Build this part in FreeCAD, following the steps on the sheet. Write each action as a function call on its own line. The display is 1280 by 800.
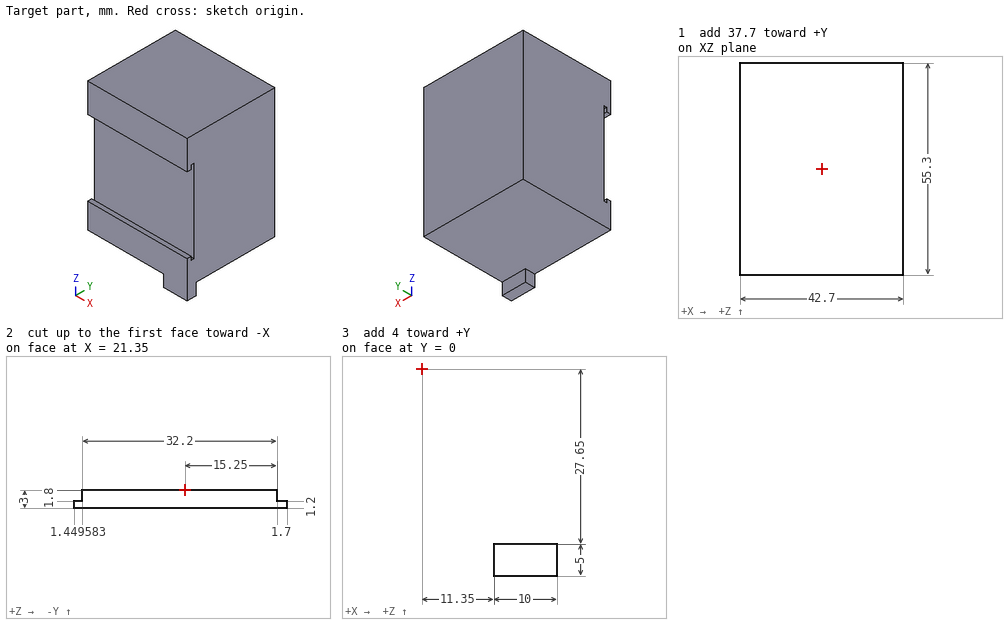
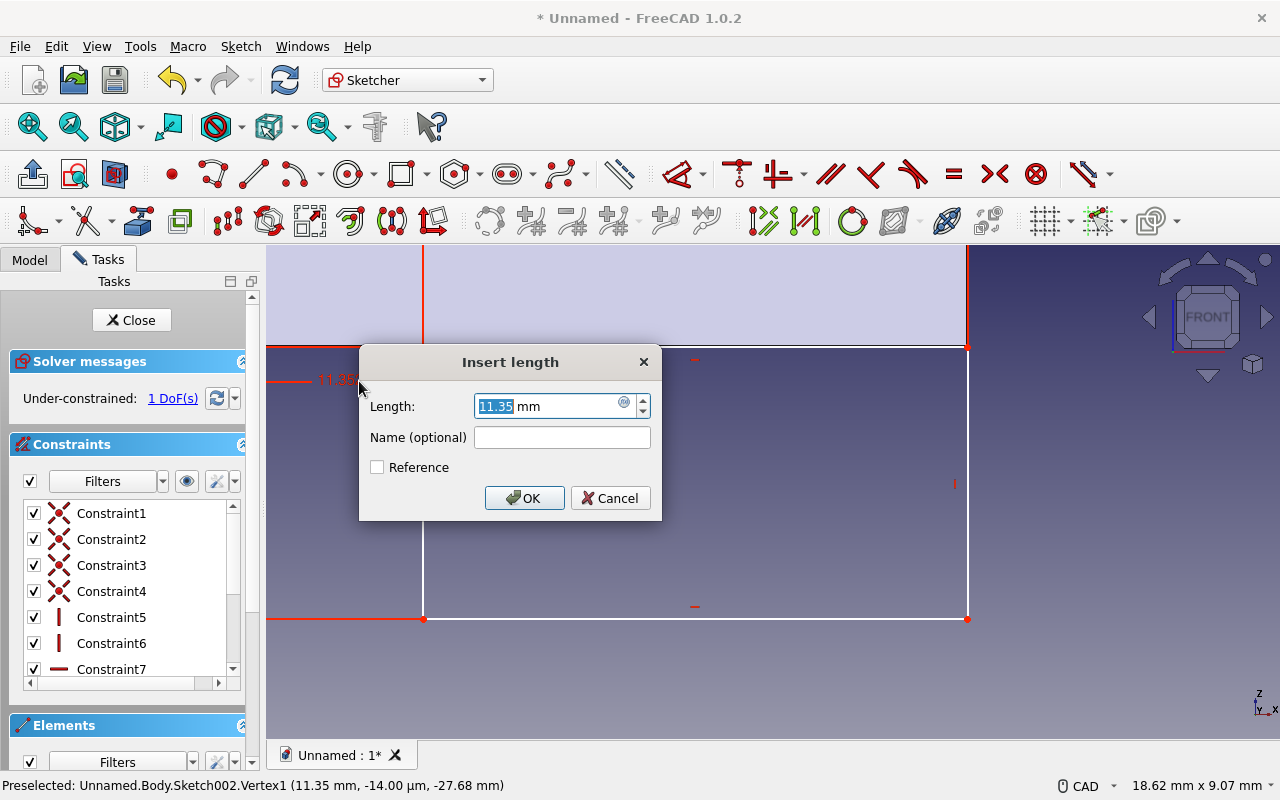
text(11.35)
key(Return)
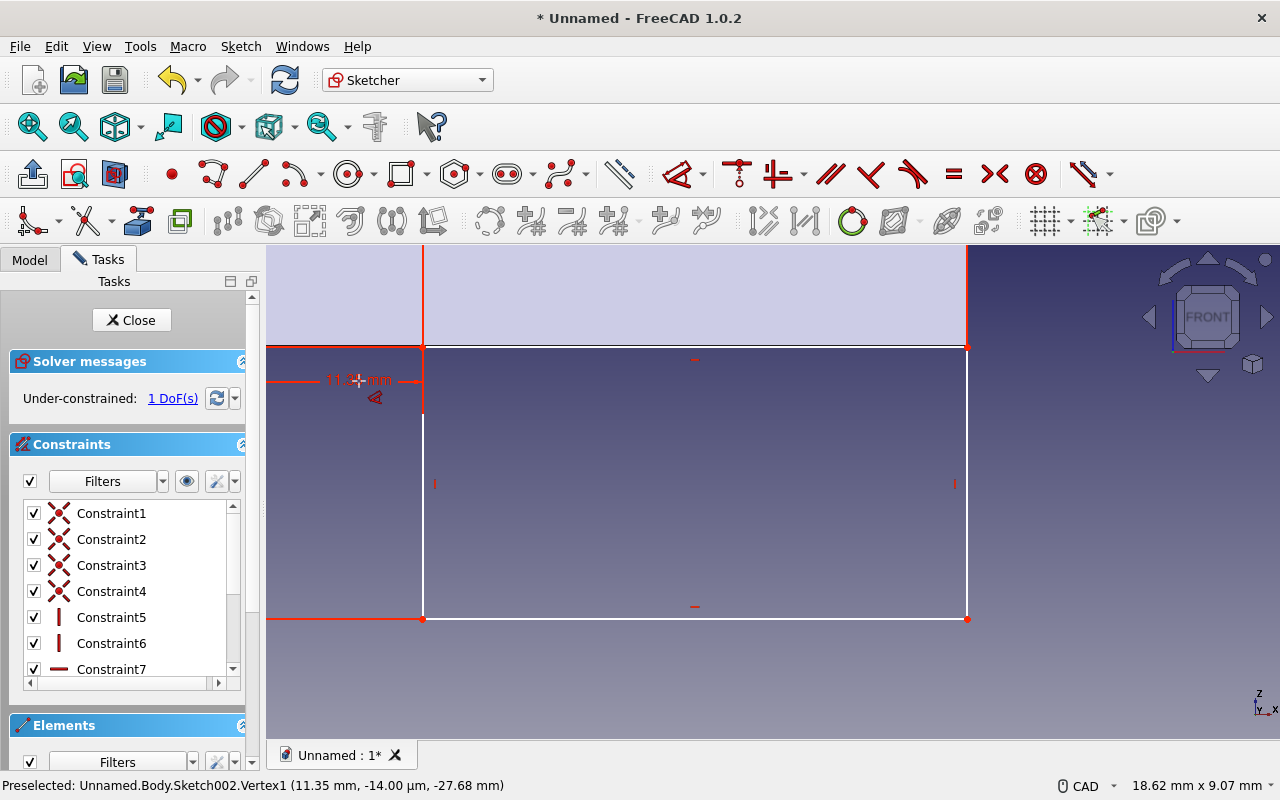
click(423, 347)
click(457, 310)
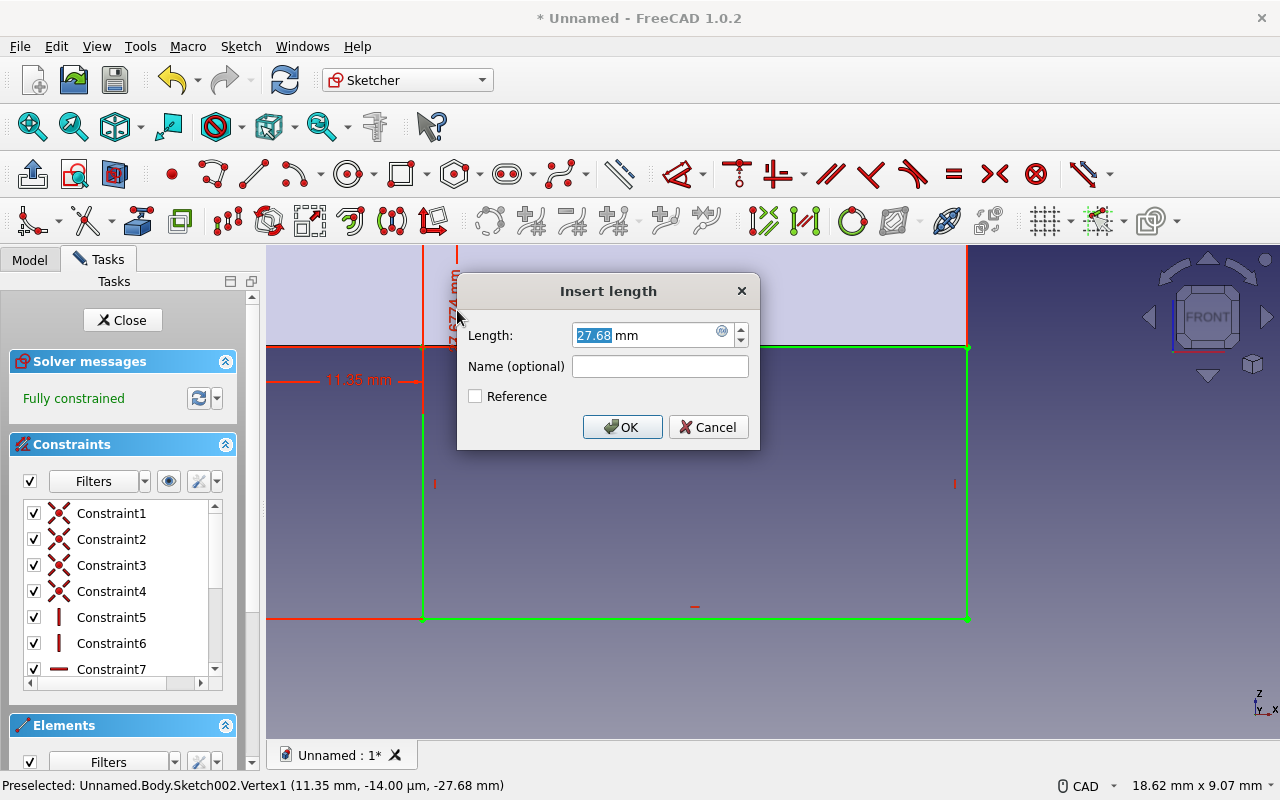
text(27.65)
key(Return)
key(Escape)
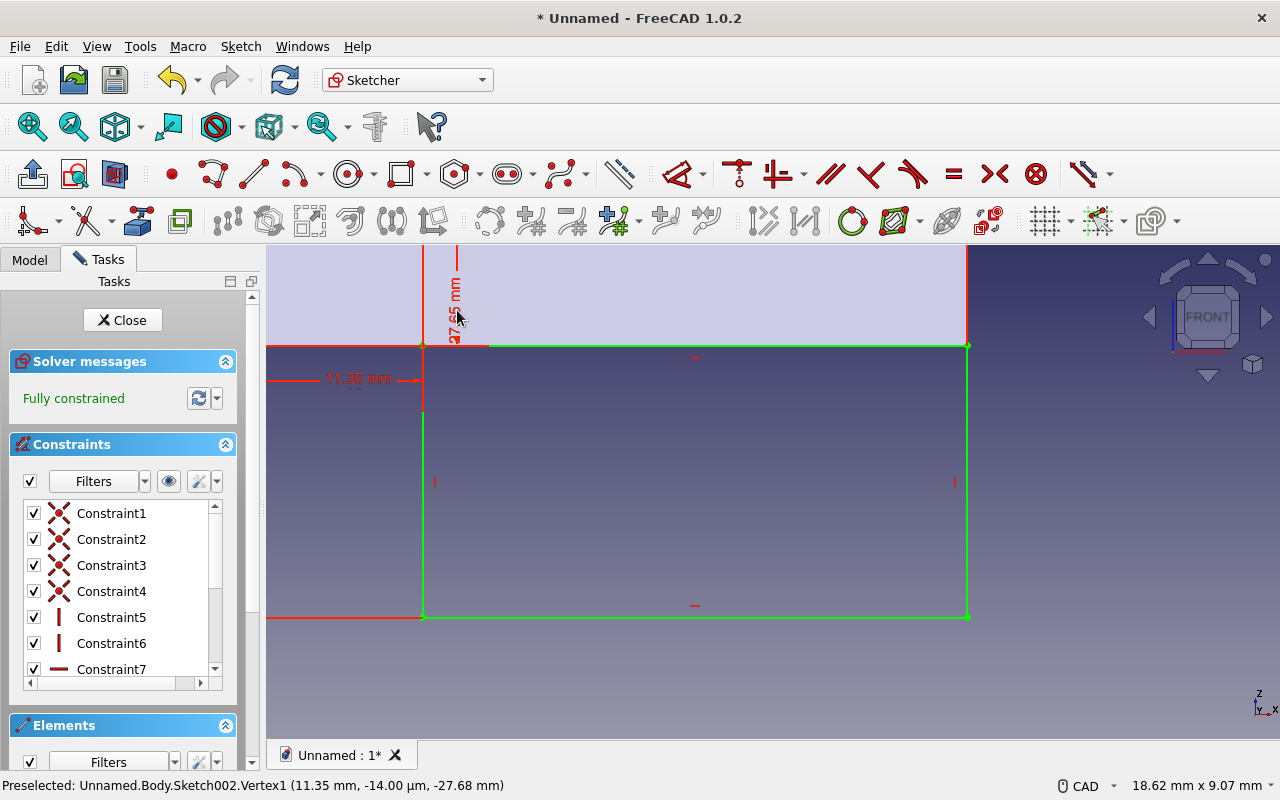
click(123, 320)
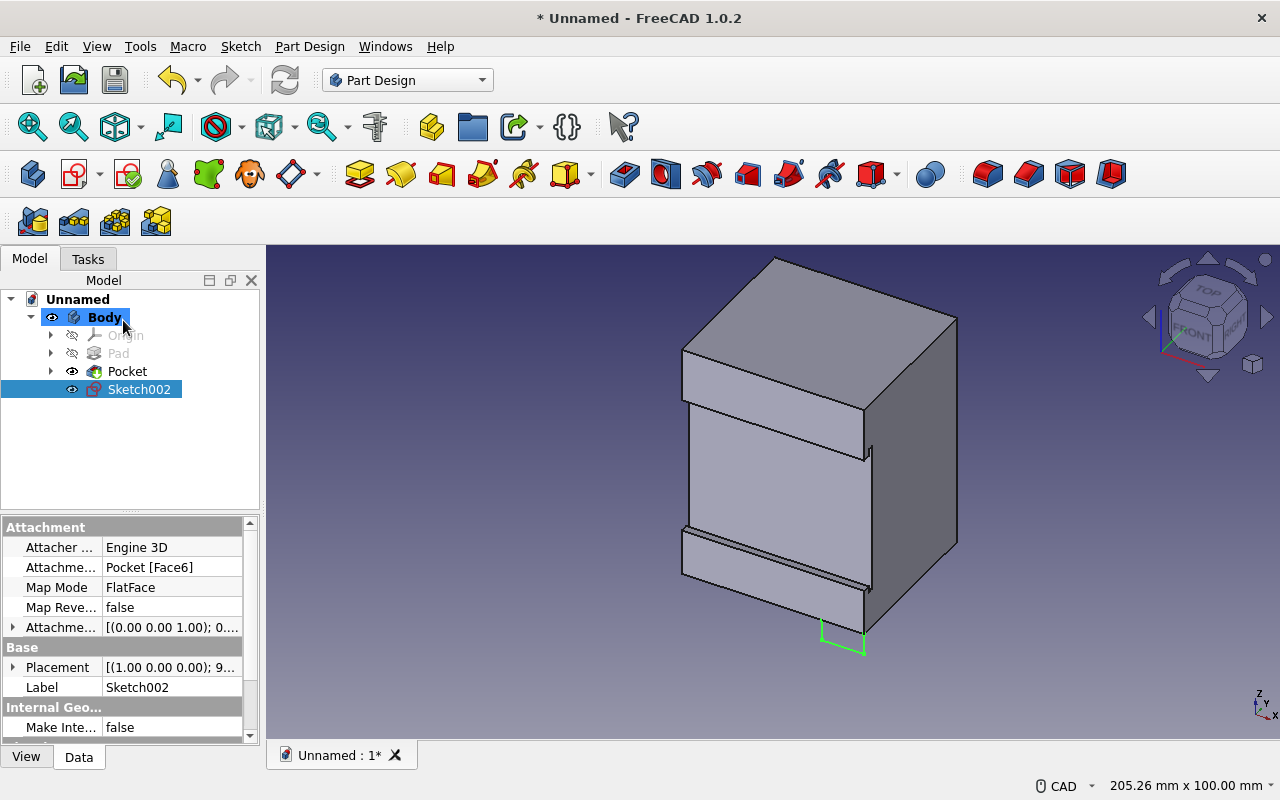
click(360, 174)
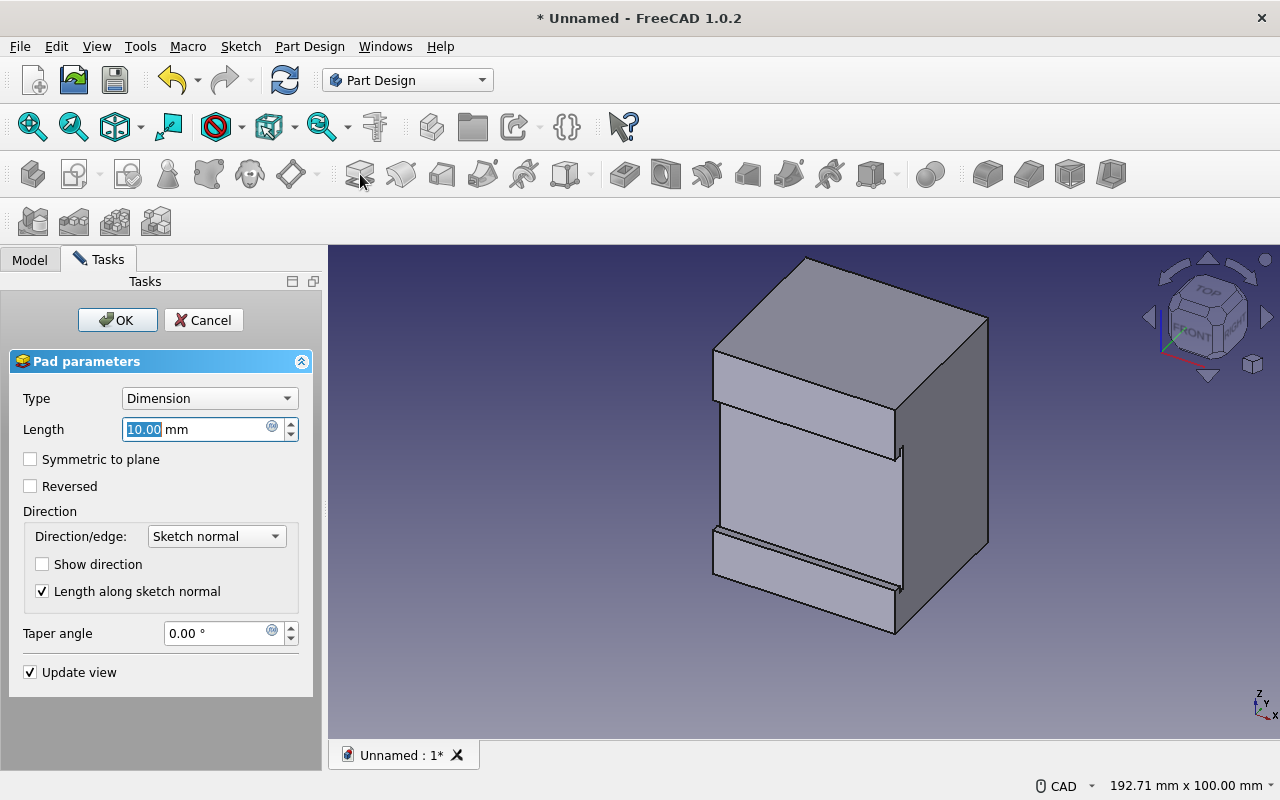
text(4)
key(Tab)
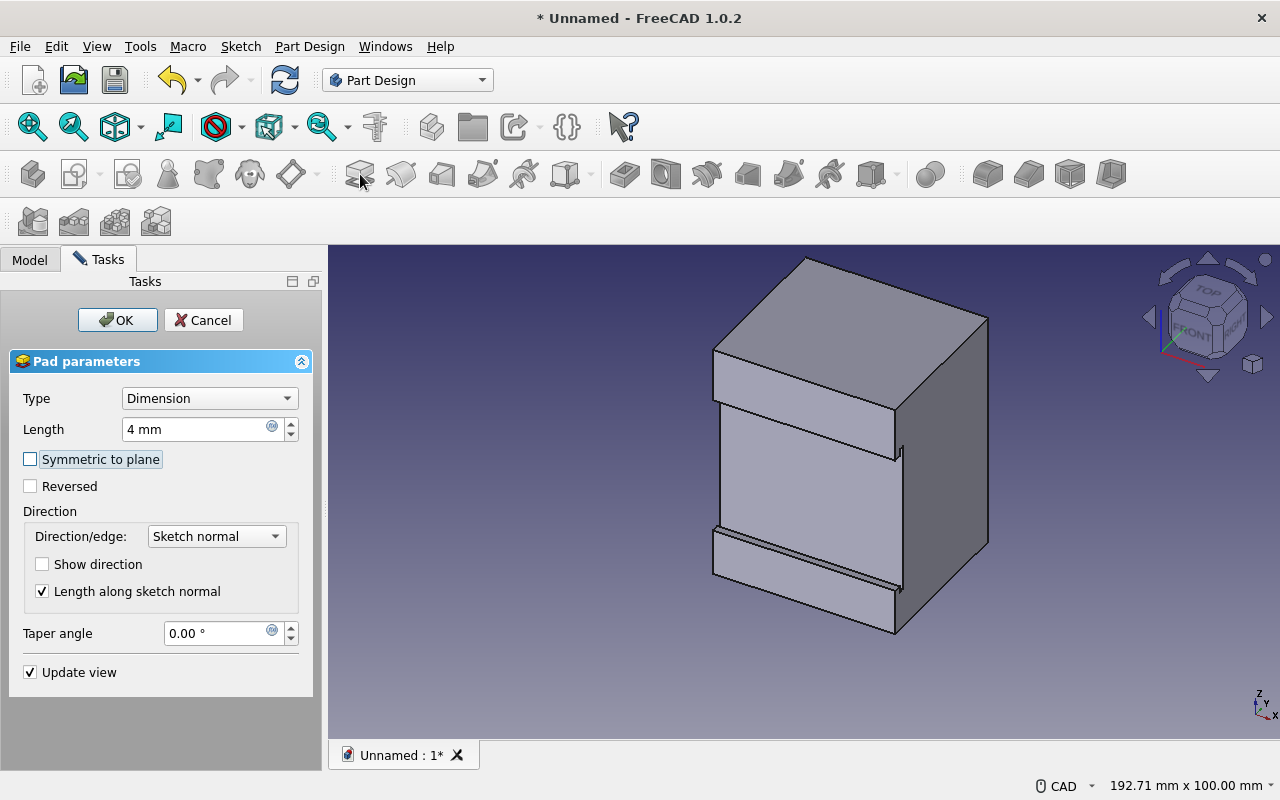
click(31, 486)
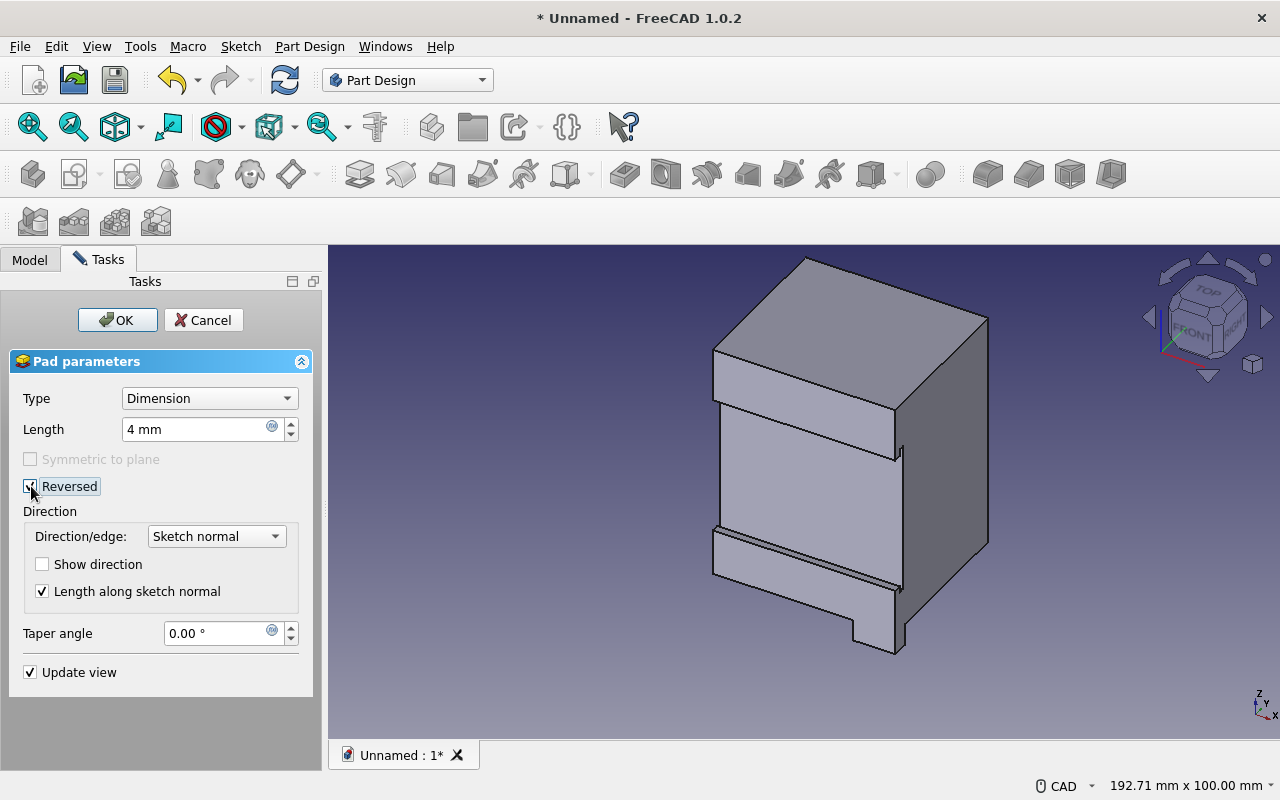
click(118, 320)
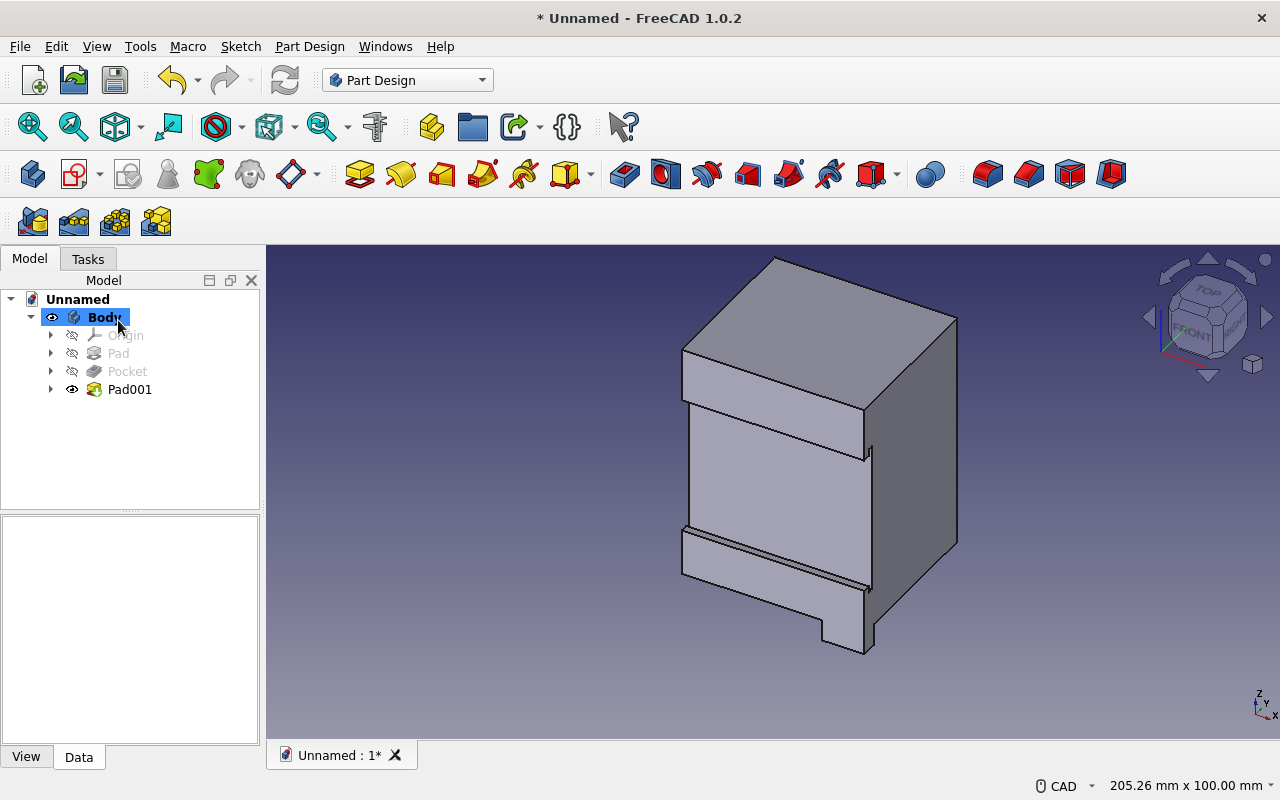
key(0)